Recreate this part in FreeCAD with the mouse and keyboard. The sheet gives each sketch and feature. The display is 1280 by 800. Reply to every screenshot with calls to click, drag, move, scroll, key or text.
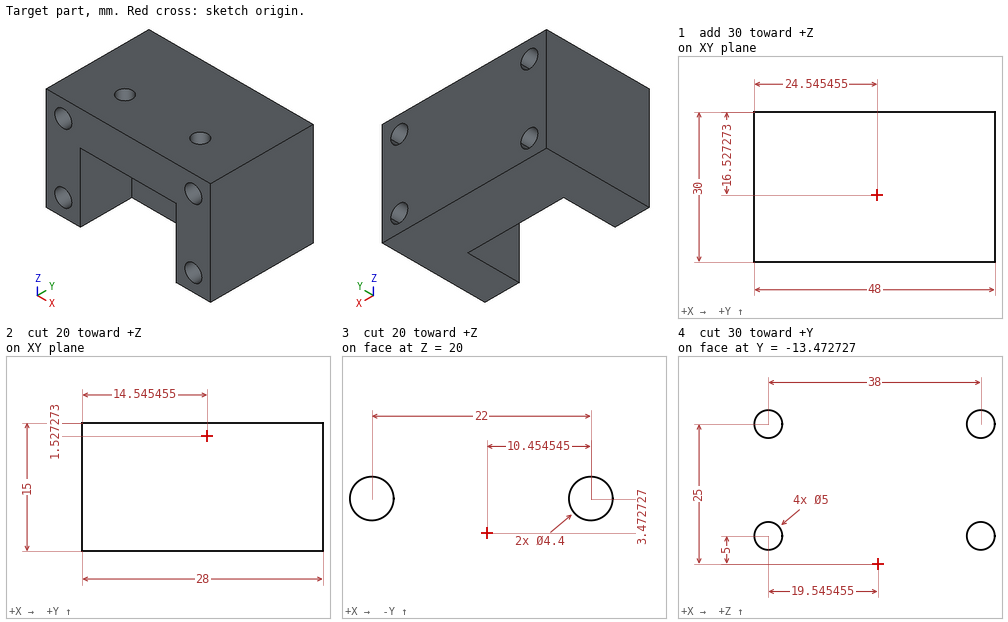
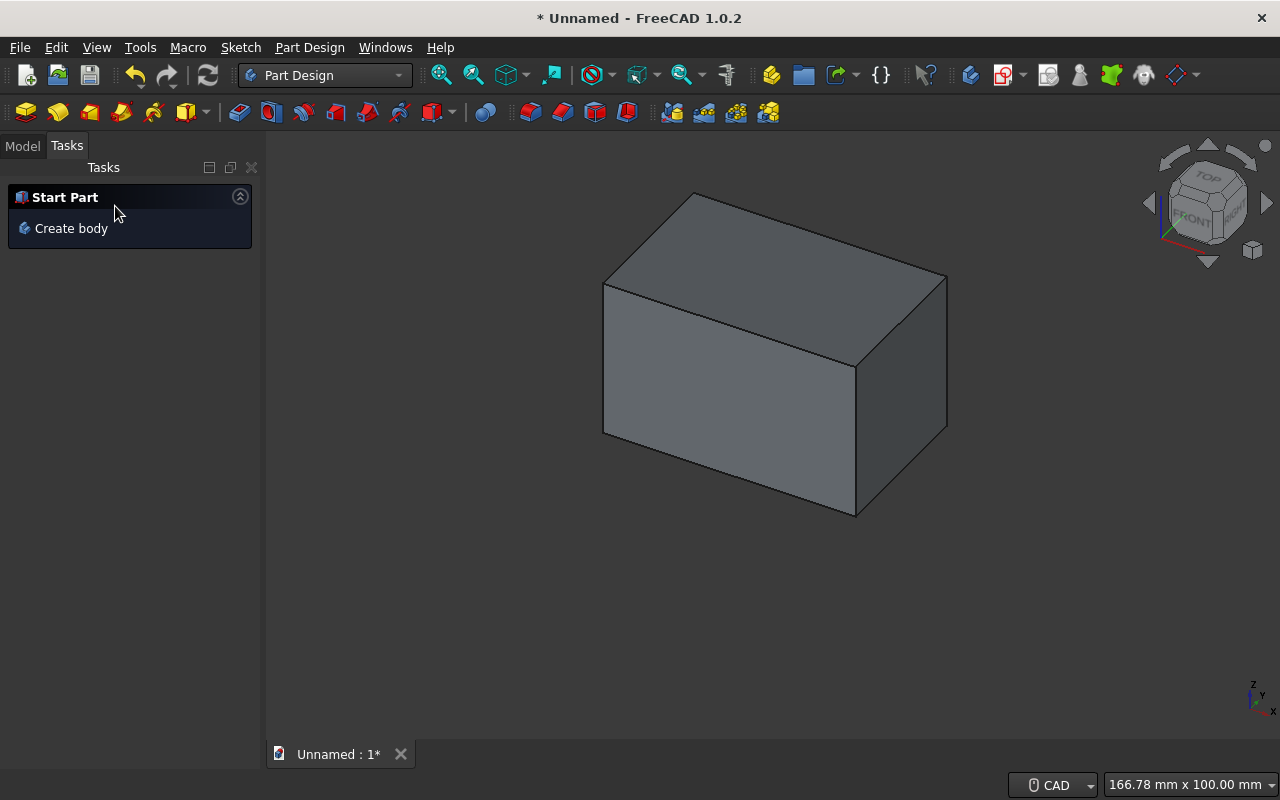
click(1004, 76)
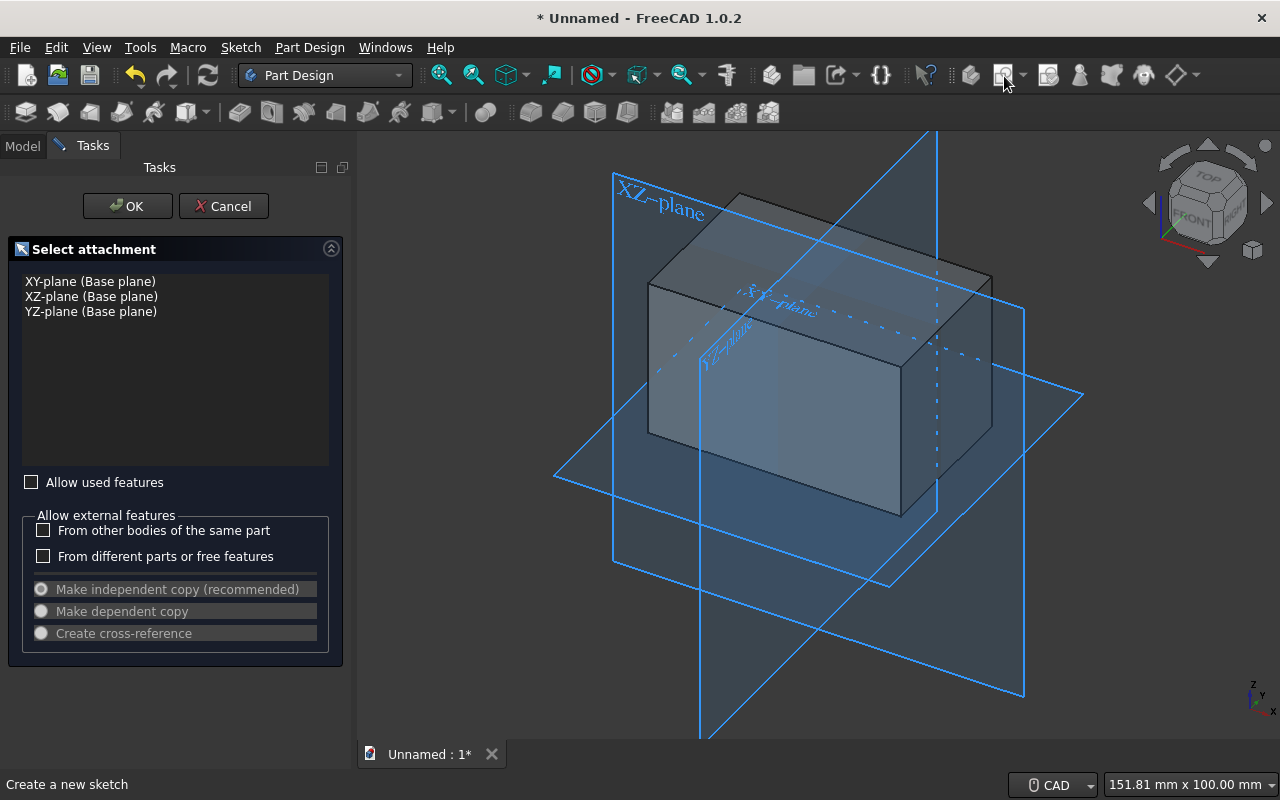
click(82, 282)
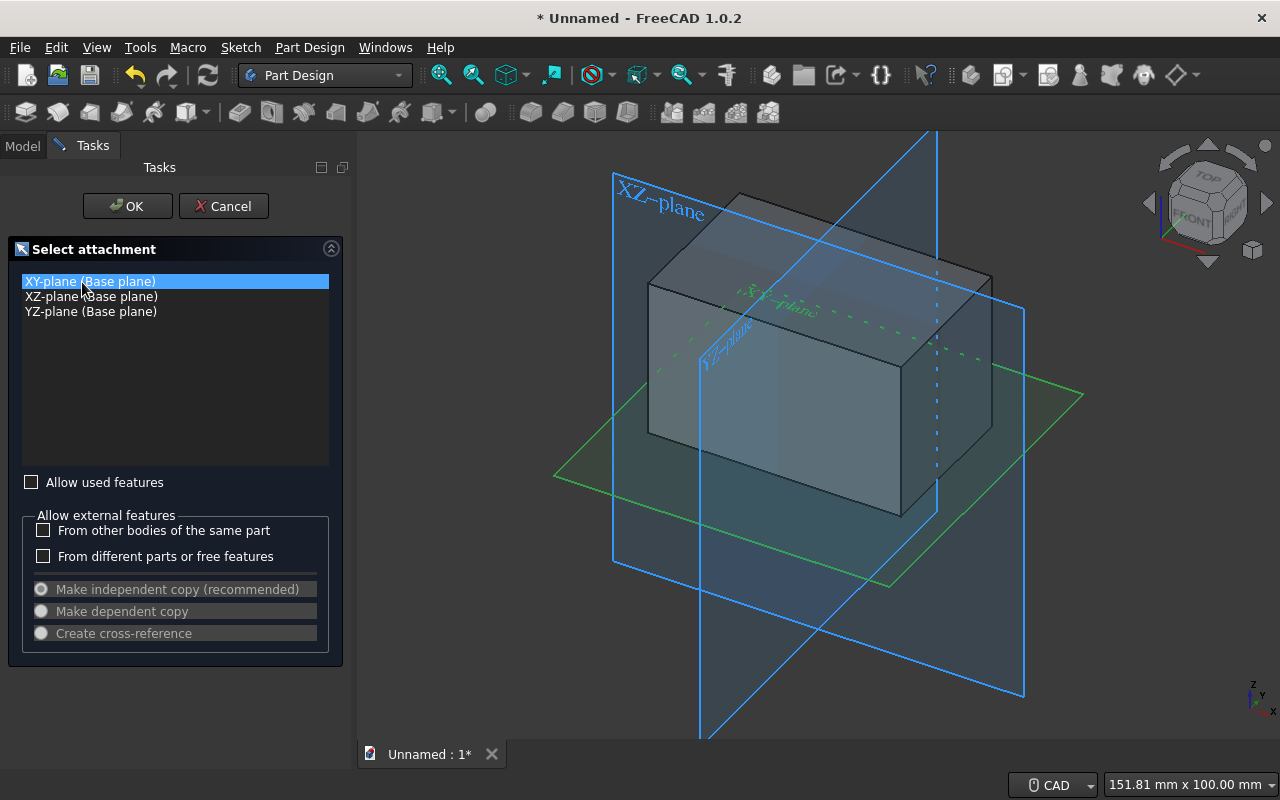
click(128, 206)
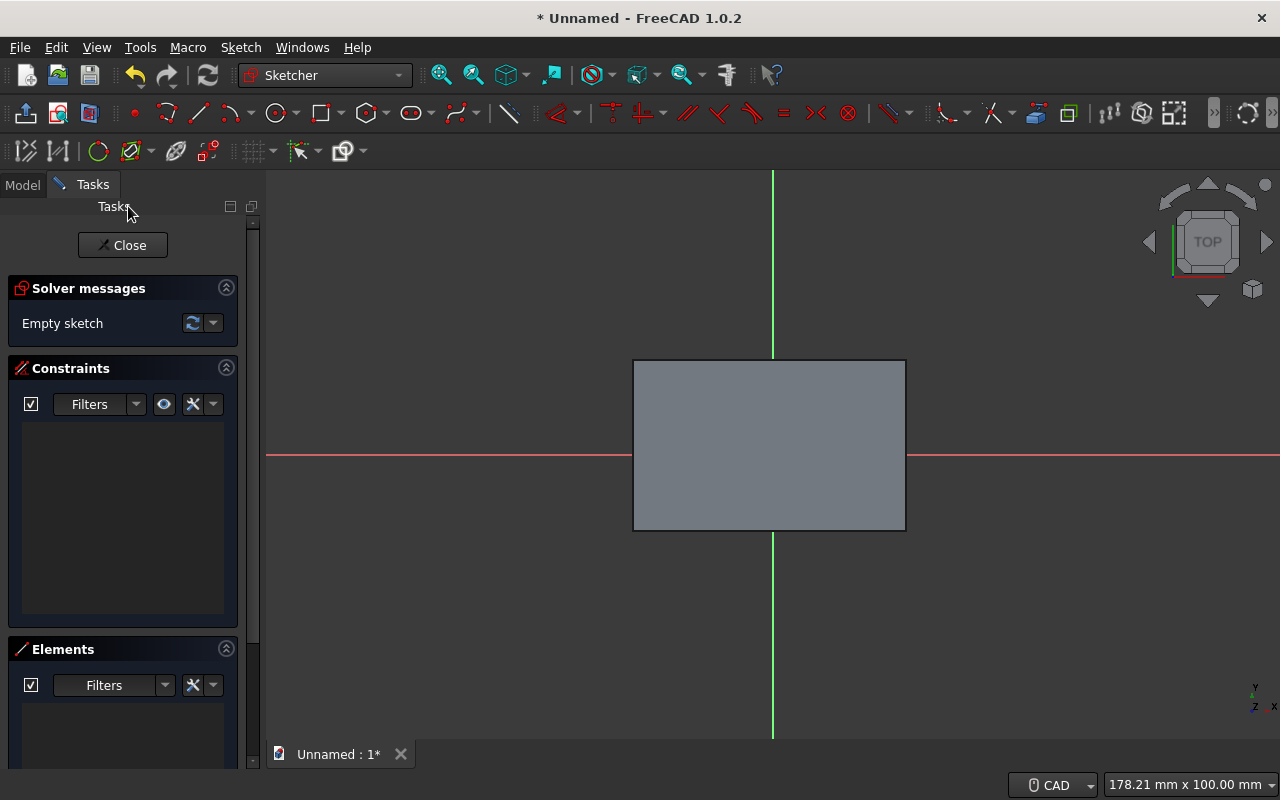
click(90, 114)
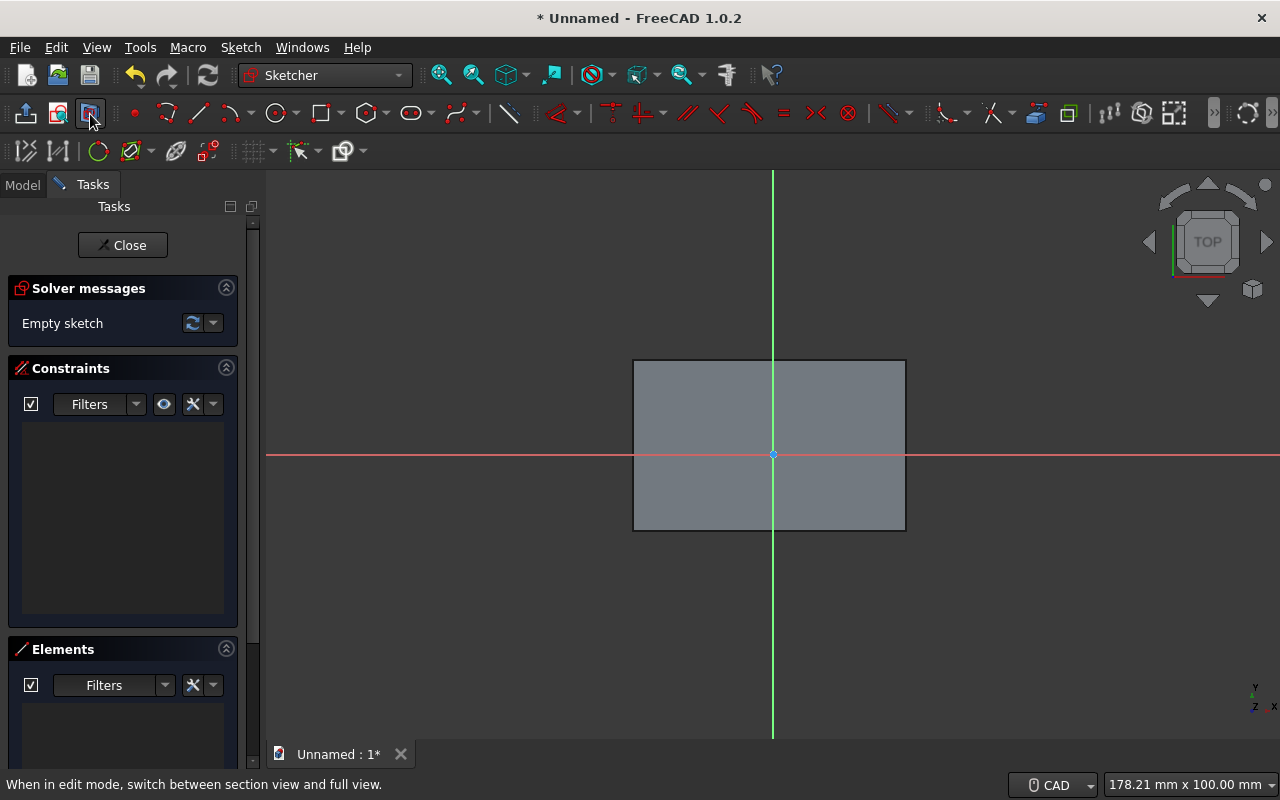
scroll(798, 503, up, 6)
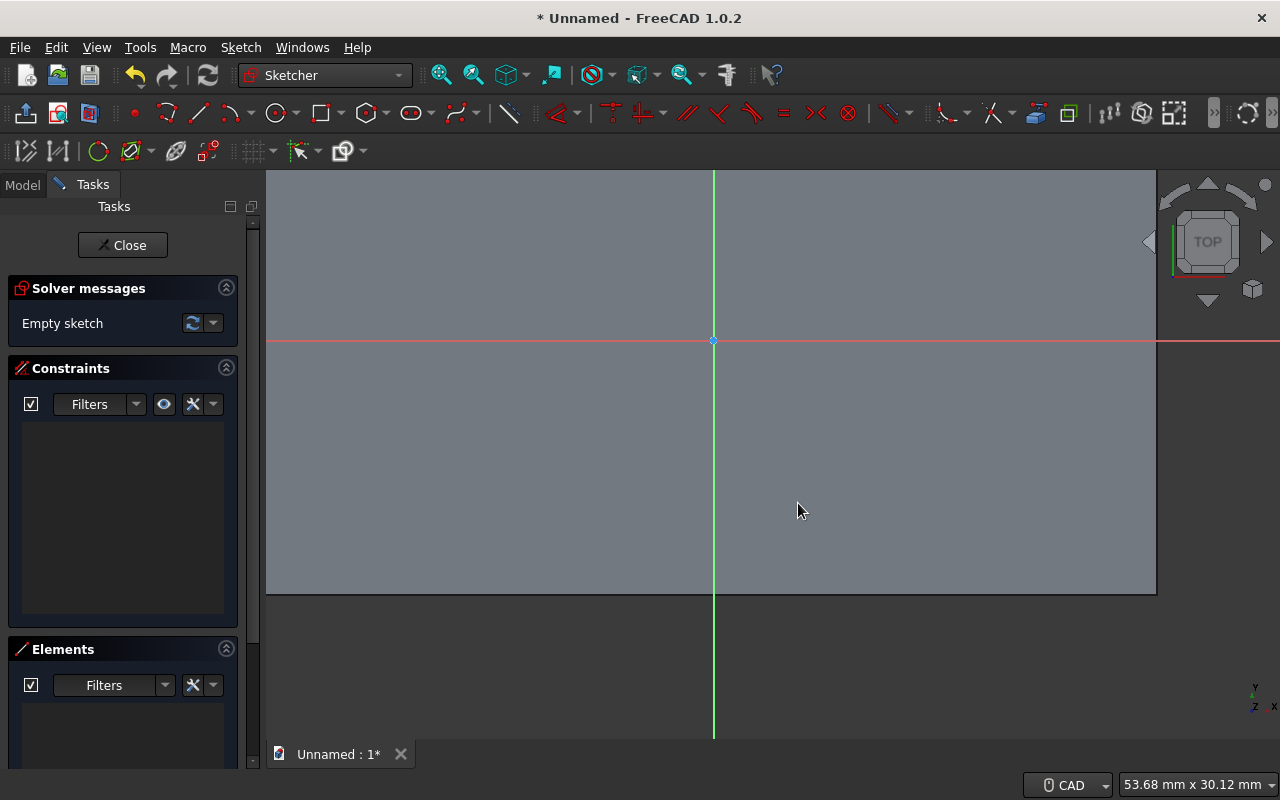
click(322, 114)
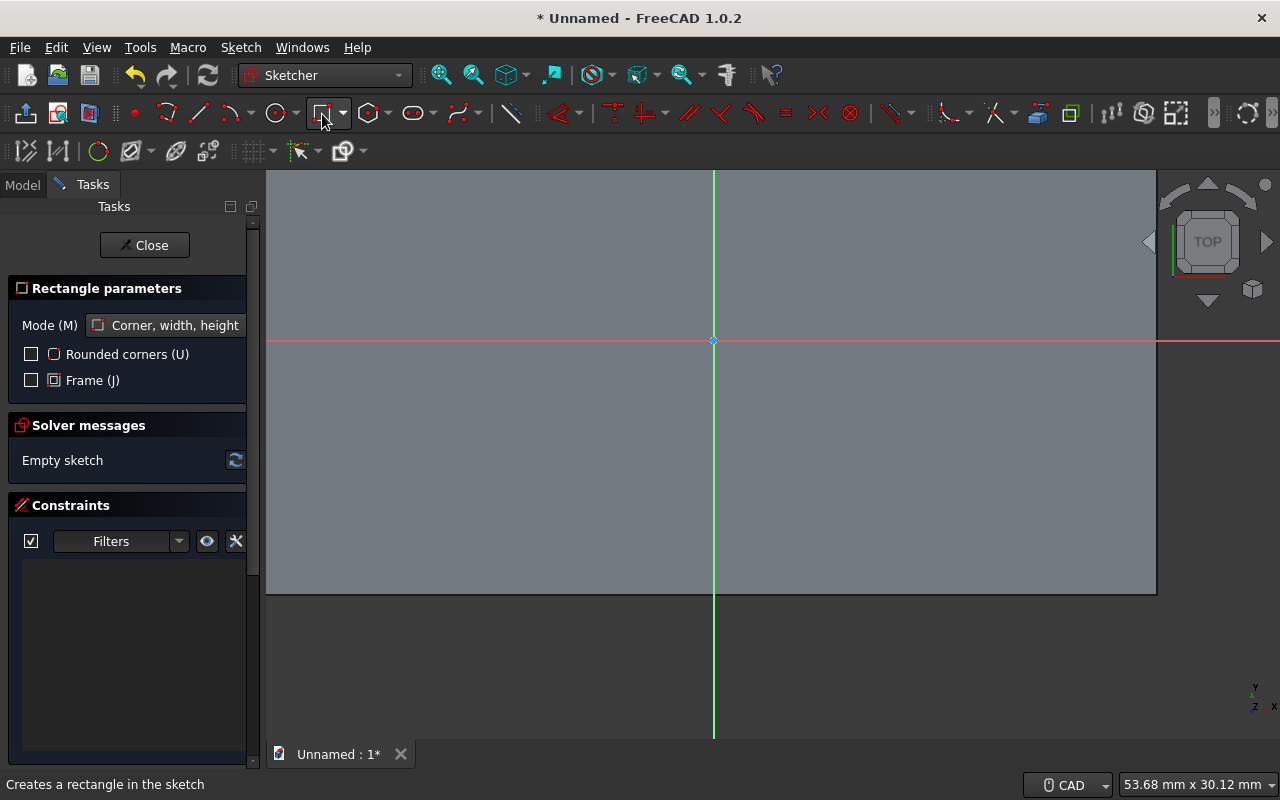
click(439, 312)
click(968, 595)
key(Escape)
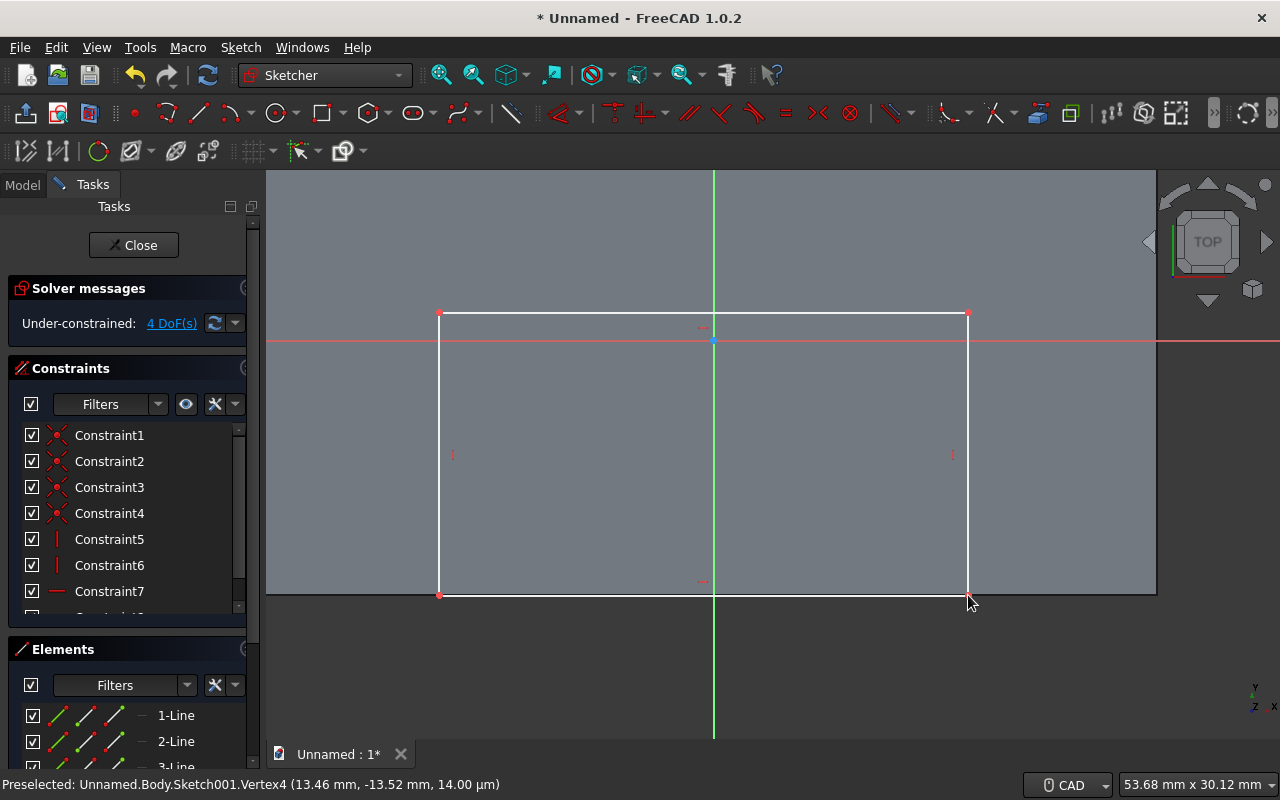
click(558, 114)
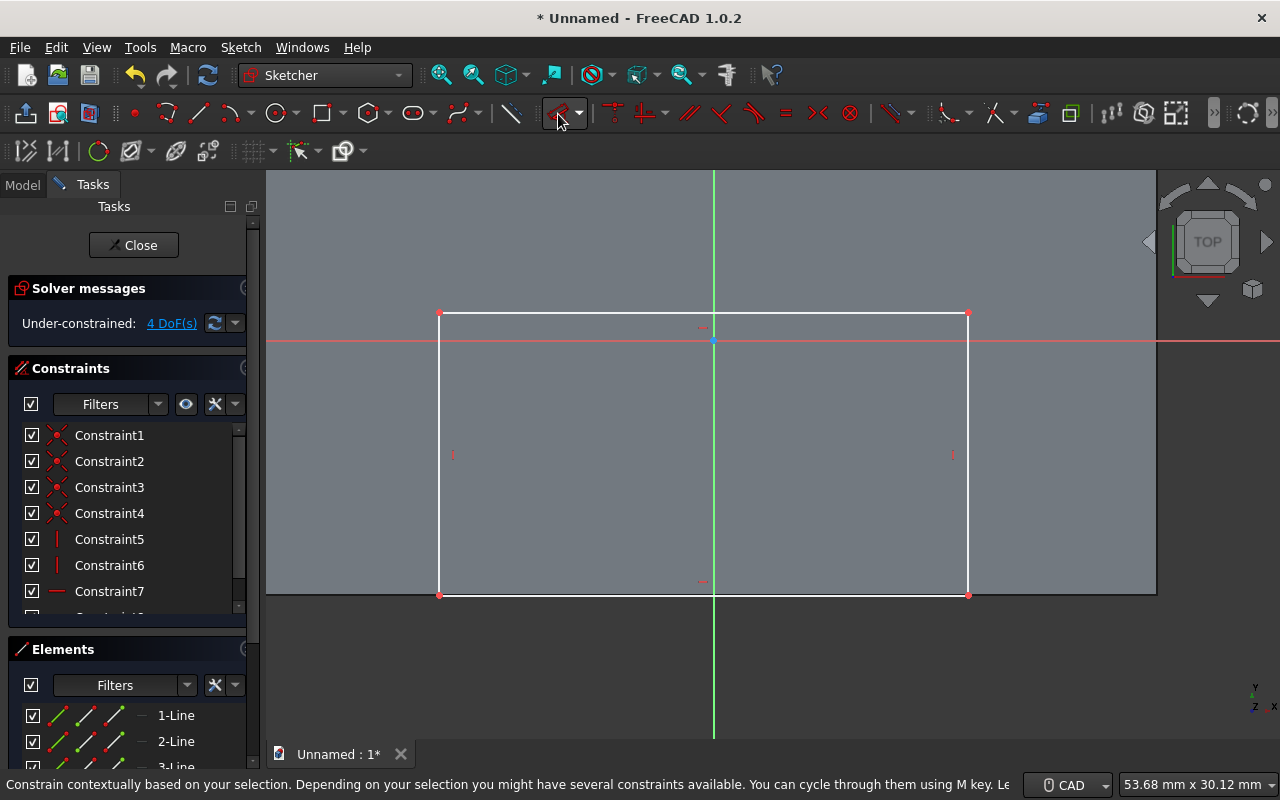
click(439, 398)
click(405, 455)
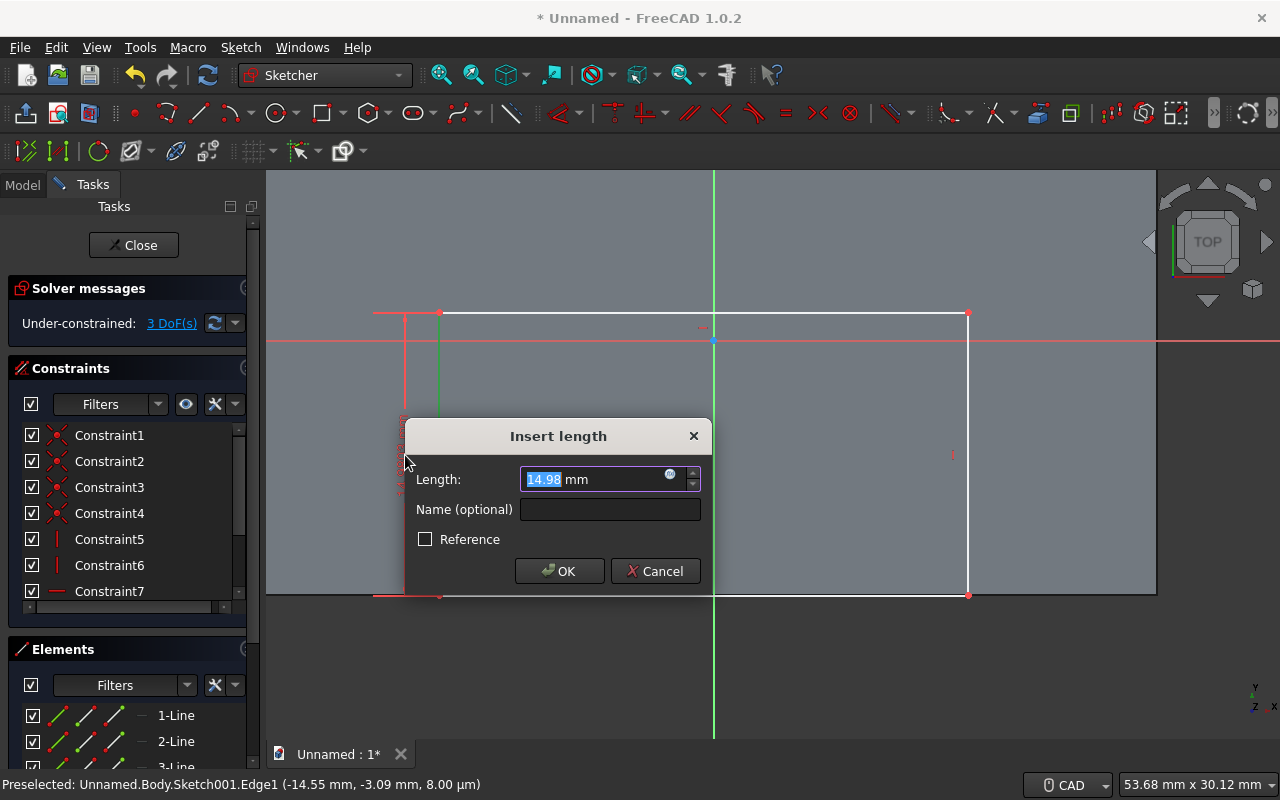
text(15)
key(Return)